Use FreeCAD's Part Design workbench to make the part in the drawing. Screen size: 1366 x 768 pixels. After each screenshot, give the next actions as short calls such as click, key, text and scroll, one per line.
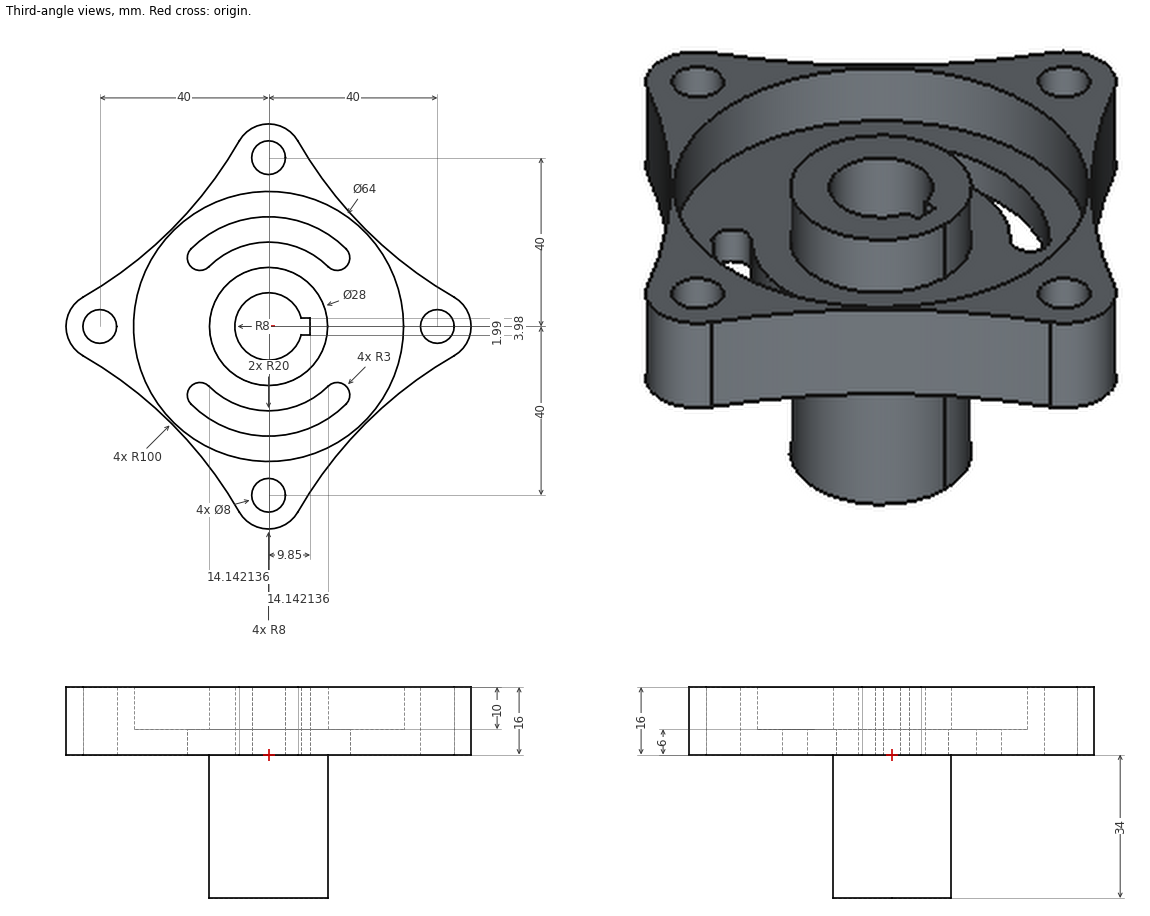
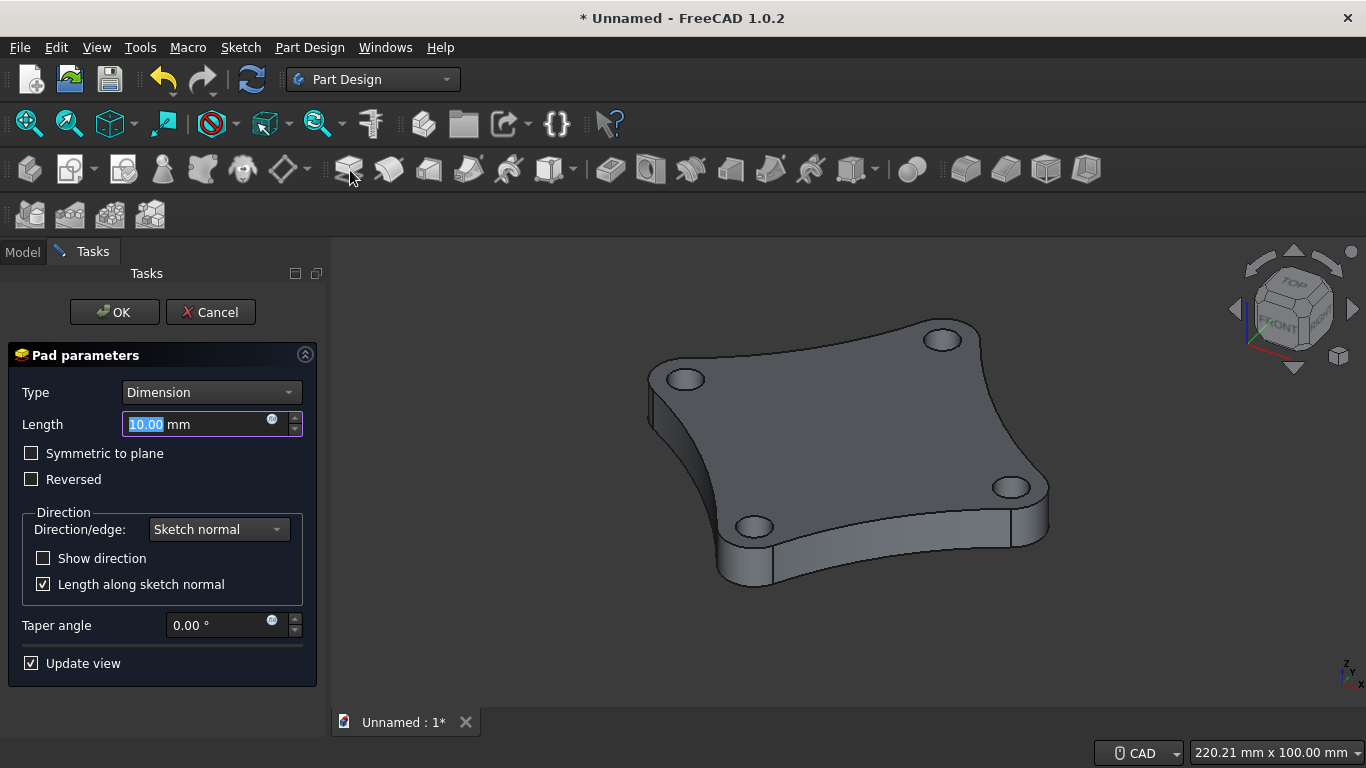
text(16)
key(Tab)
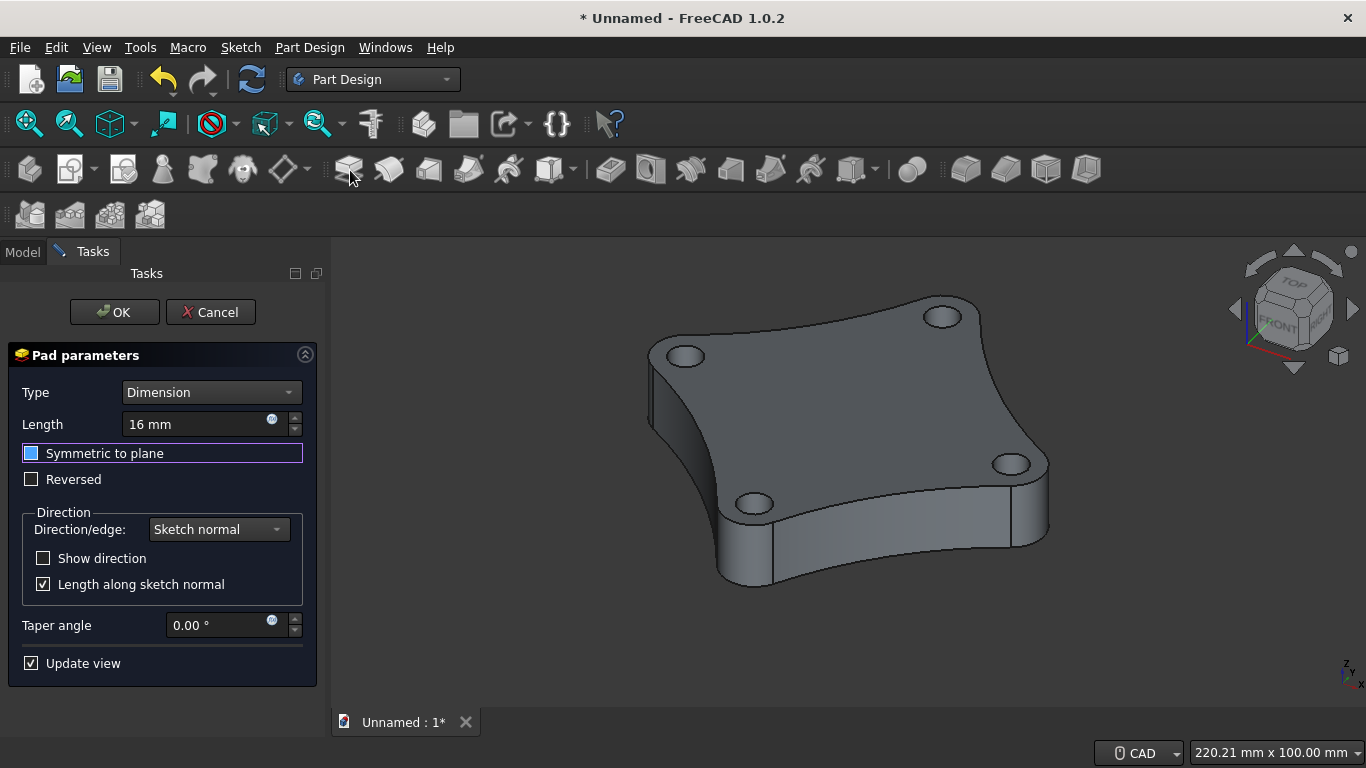
click(115, 312)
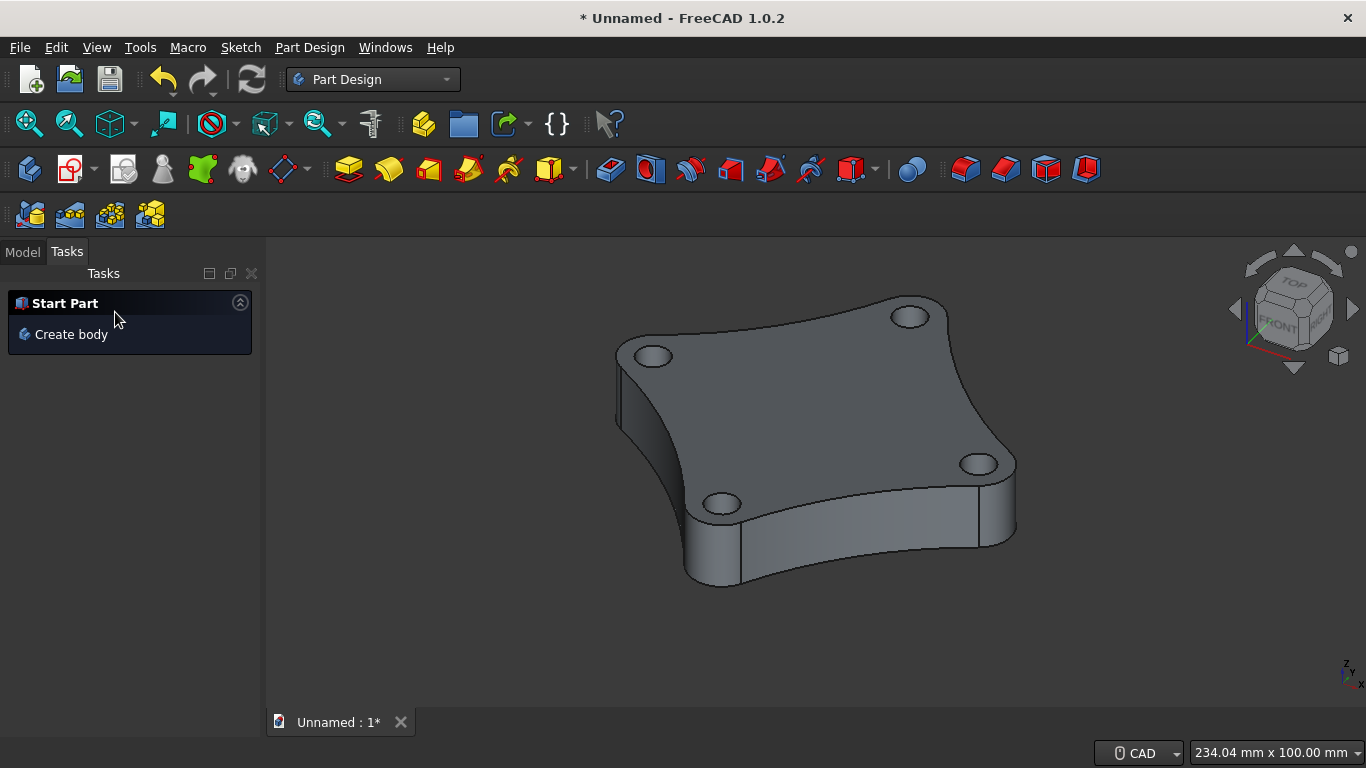
key(v)
key(f)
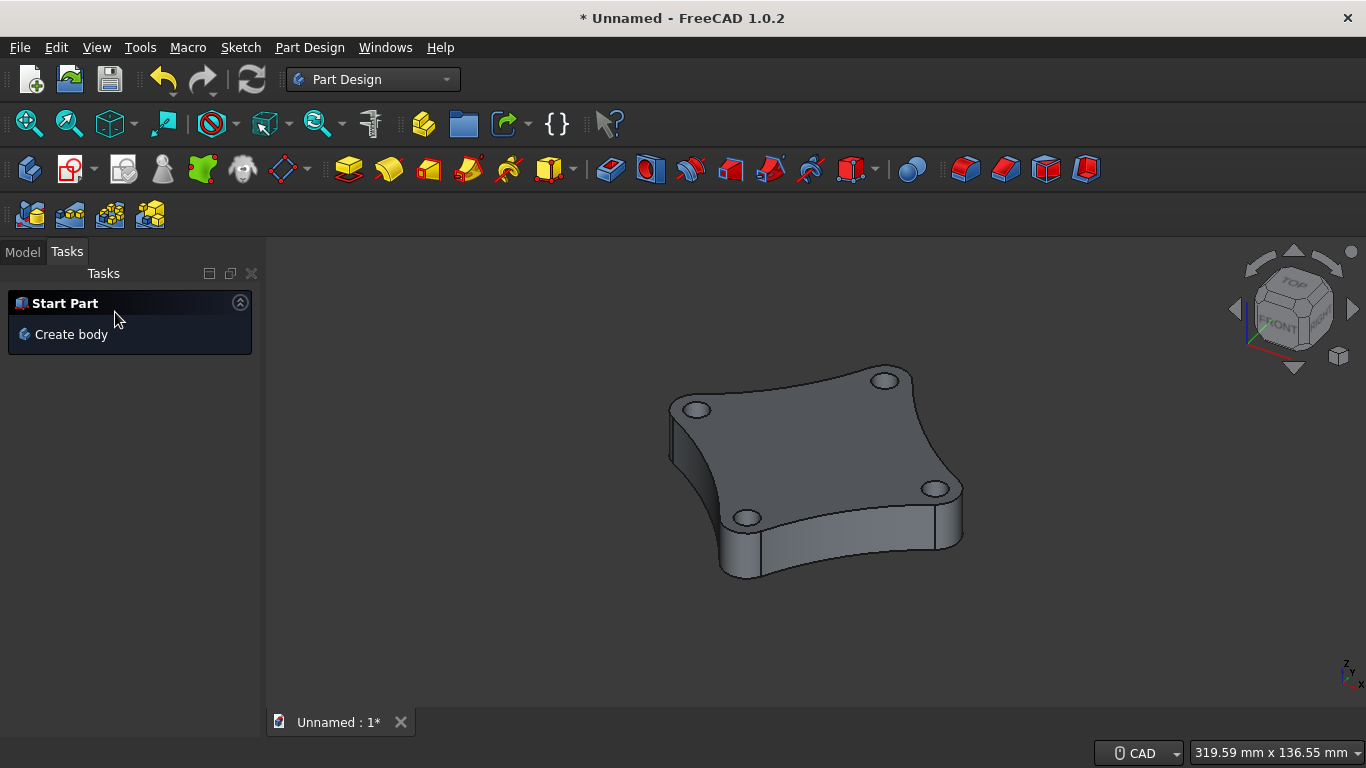
click(816, 448)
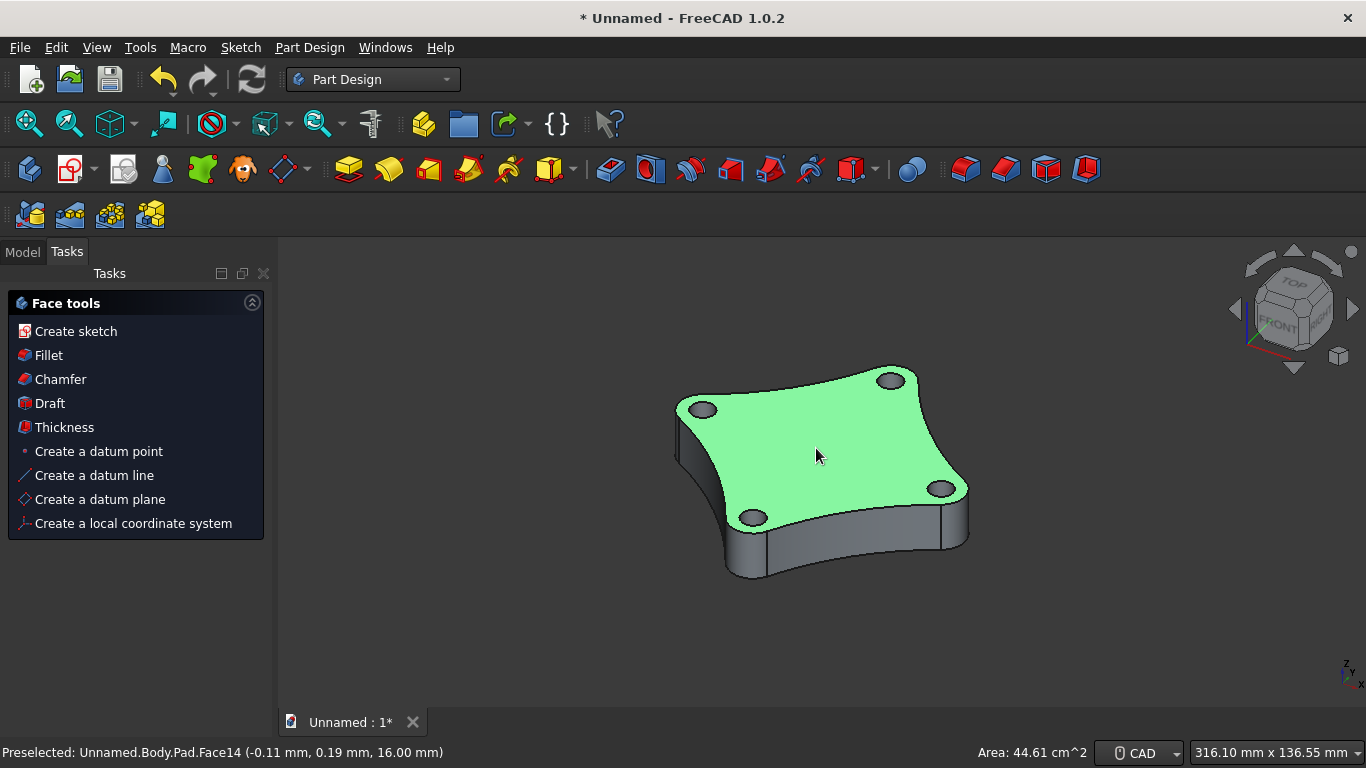
click(70, 170)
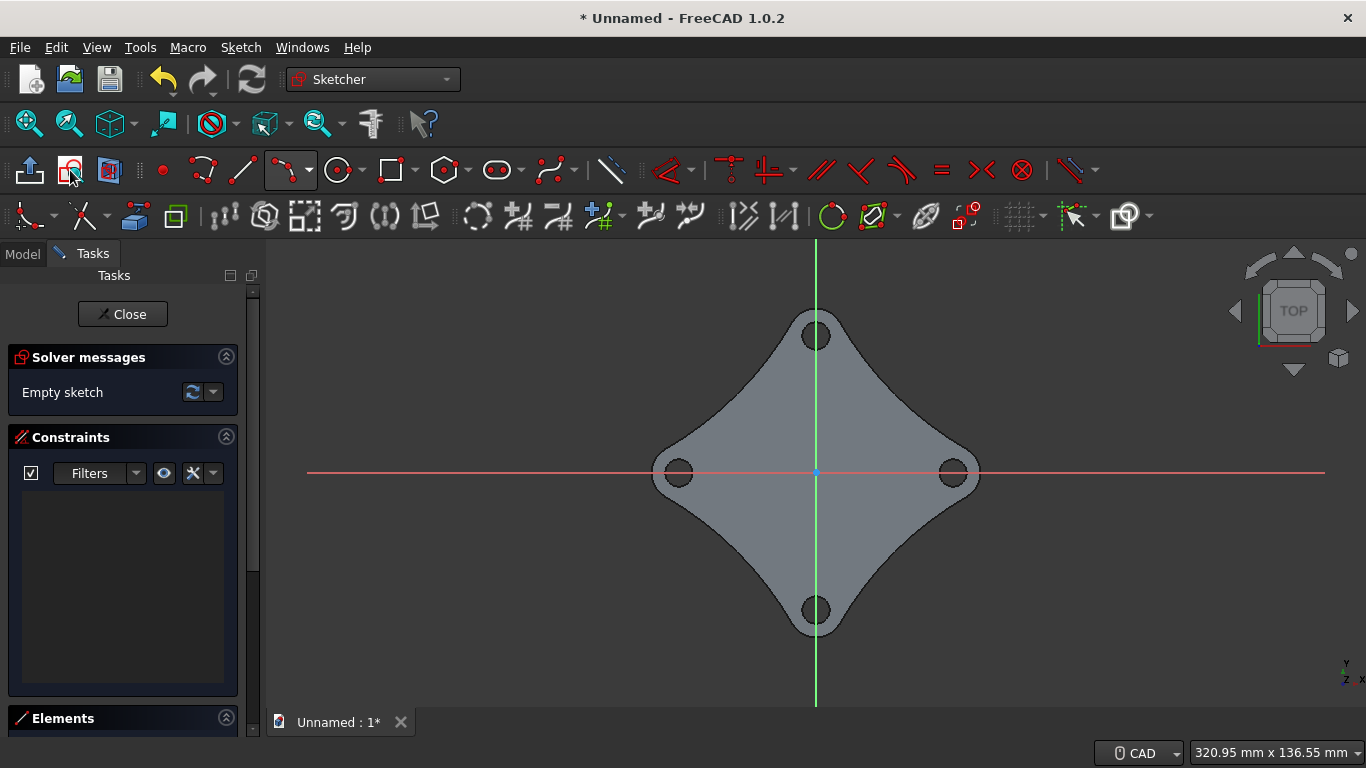
click(338, 170)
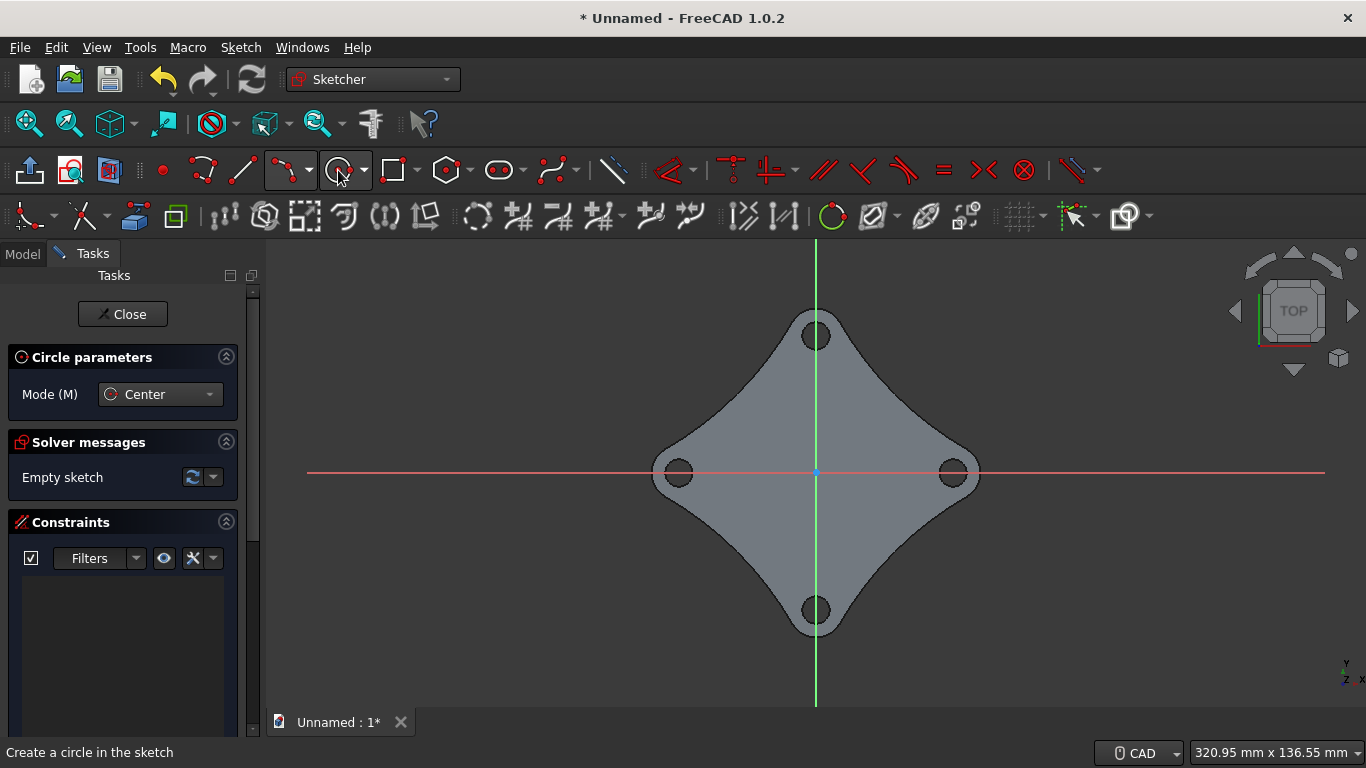
click(816, 473)
move(894, 395)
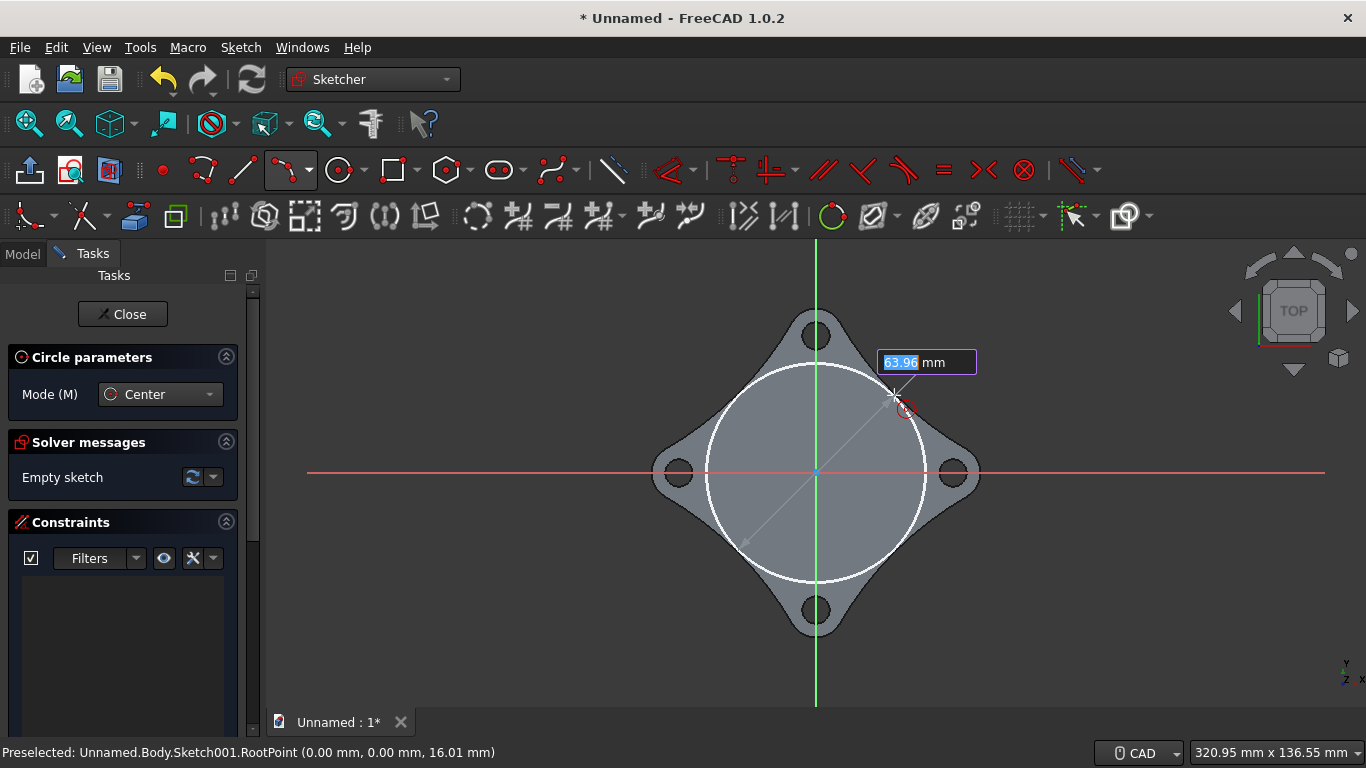
text(64)
key(Return)
key(Escape)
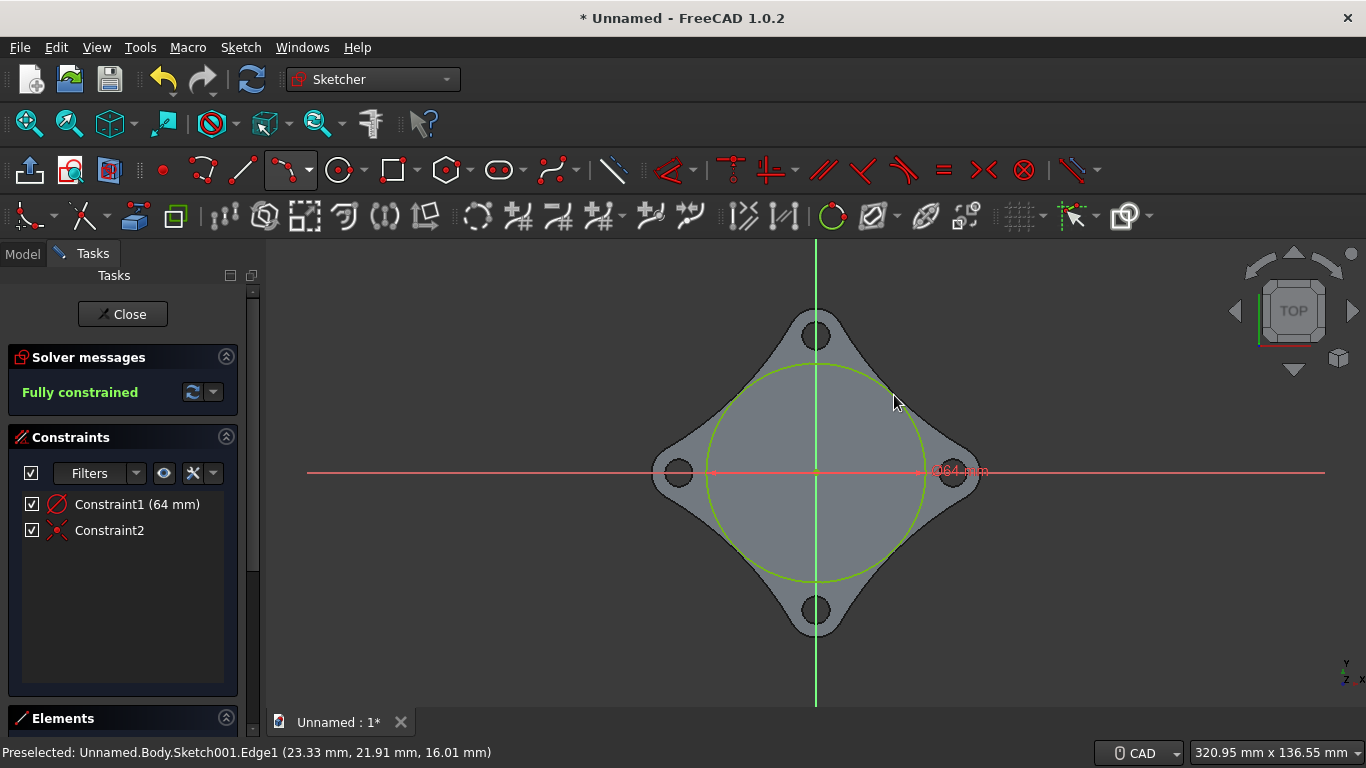
click(123, 314)